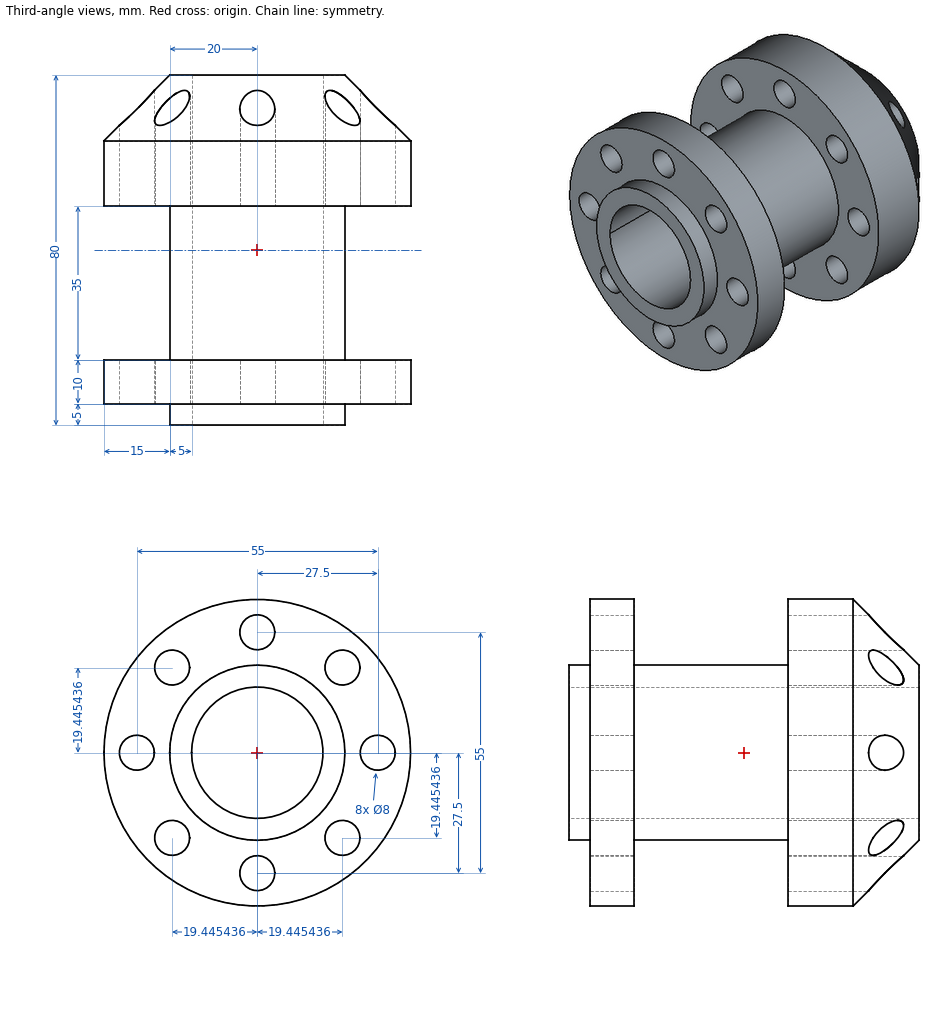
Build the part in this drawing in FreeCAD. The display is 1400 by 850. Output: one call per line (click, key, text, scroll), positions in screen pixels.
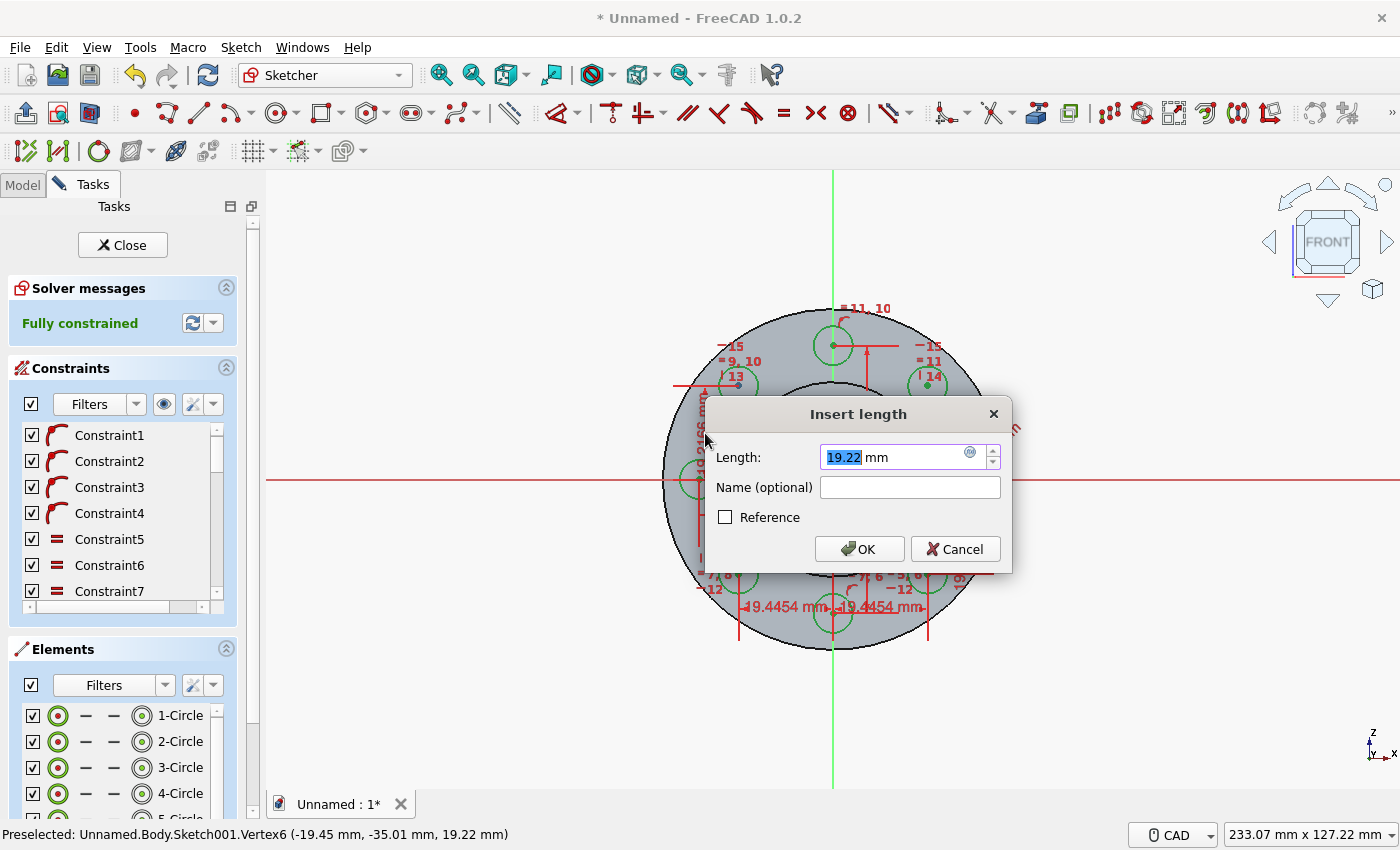
text(19.445436)
key(Return)
key(Escape)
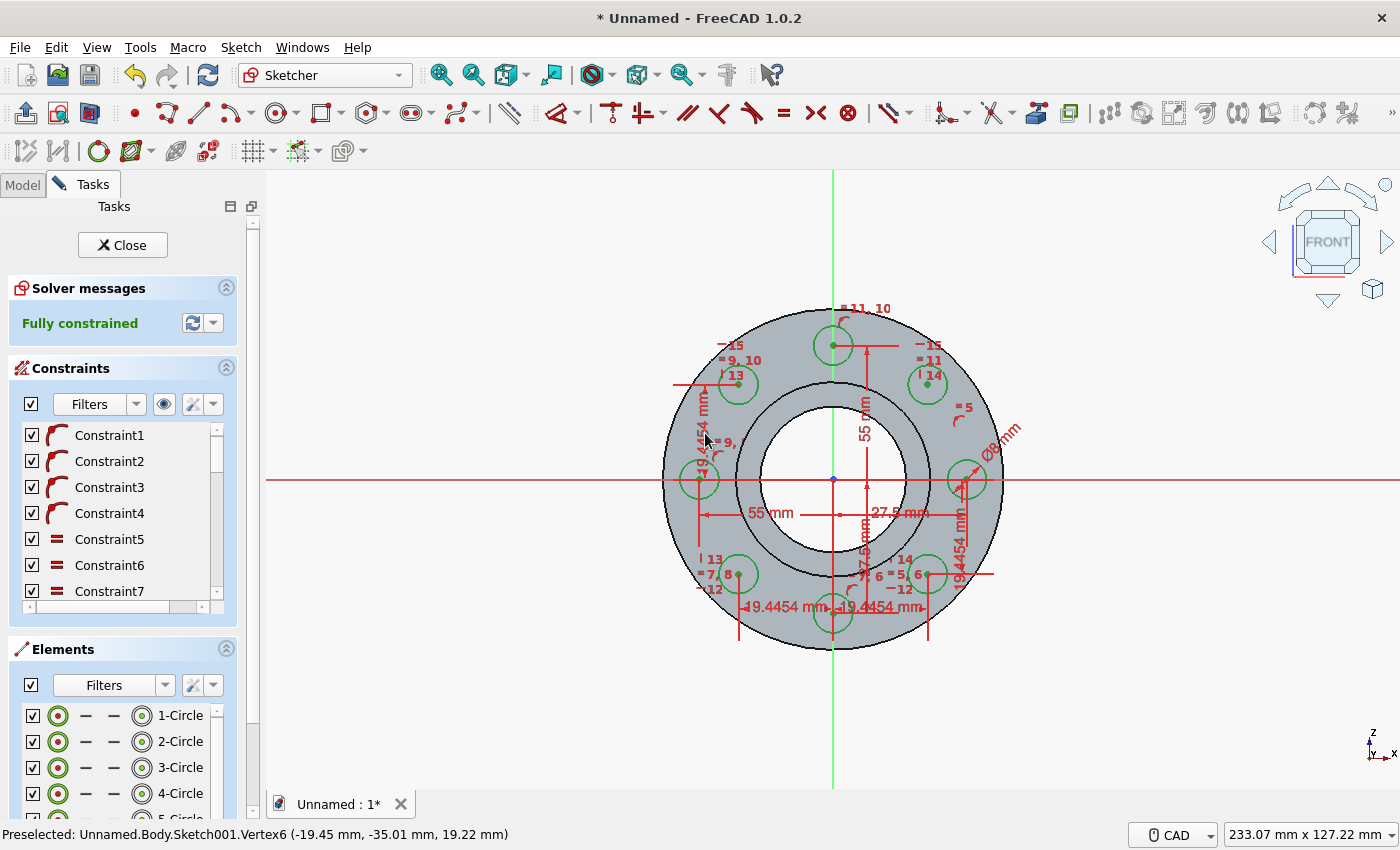
click(123, 245)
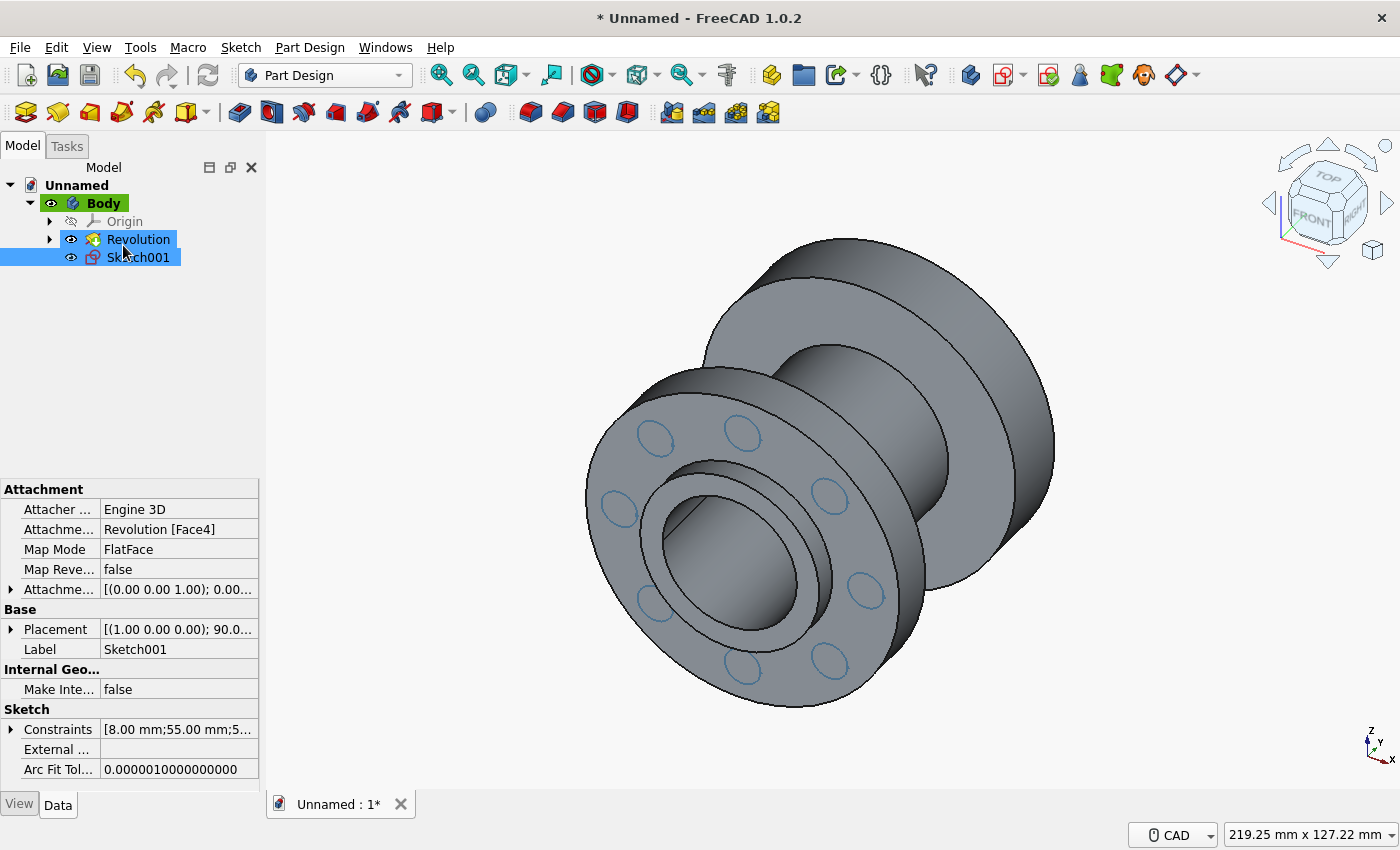
click(240, 112)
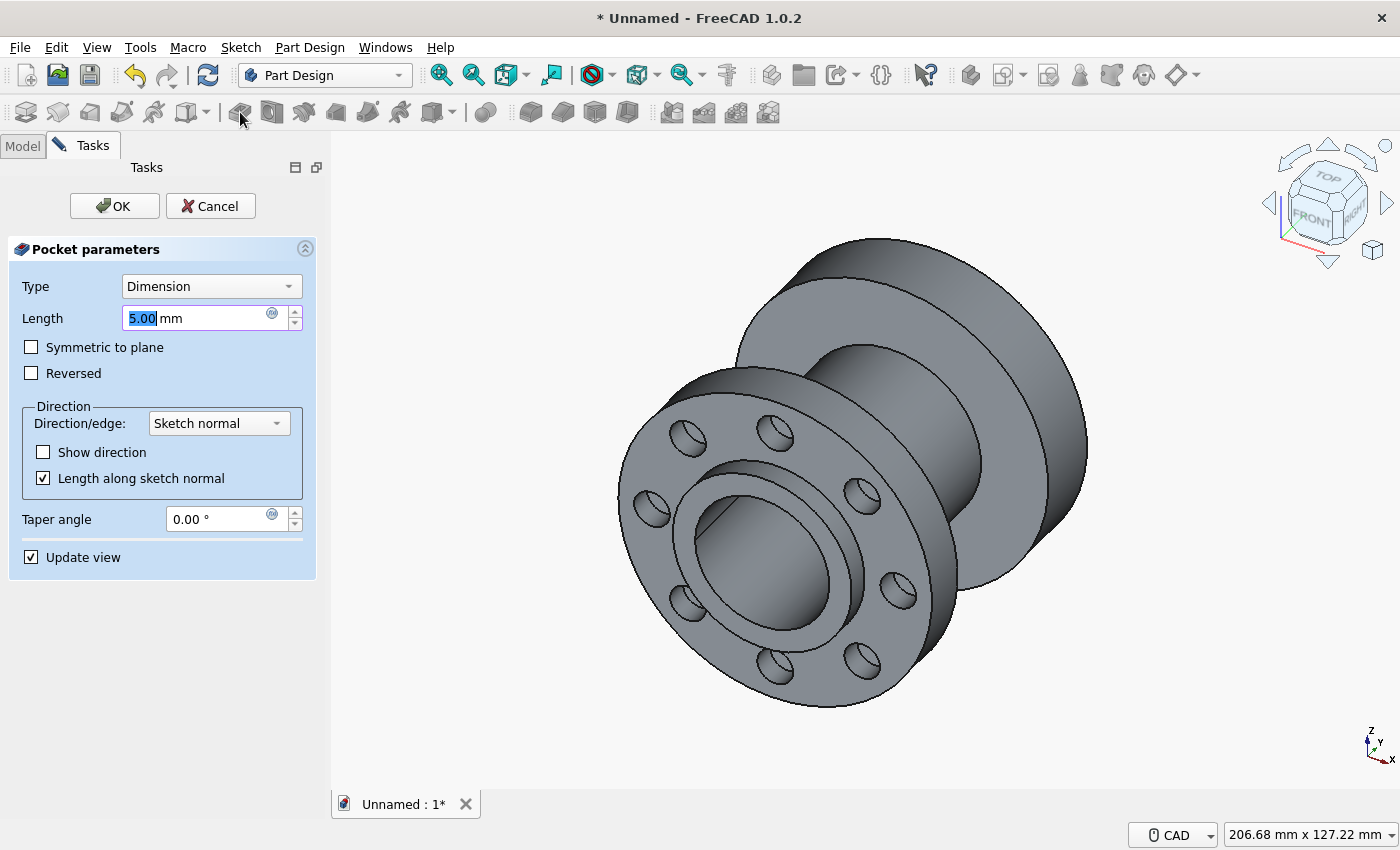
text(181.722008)
key(Tab)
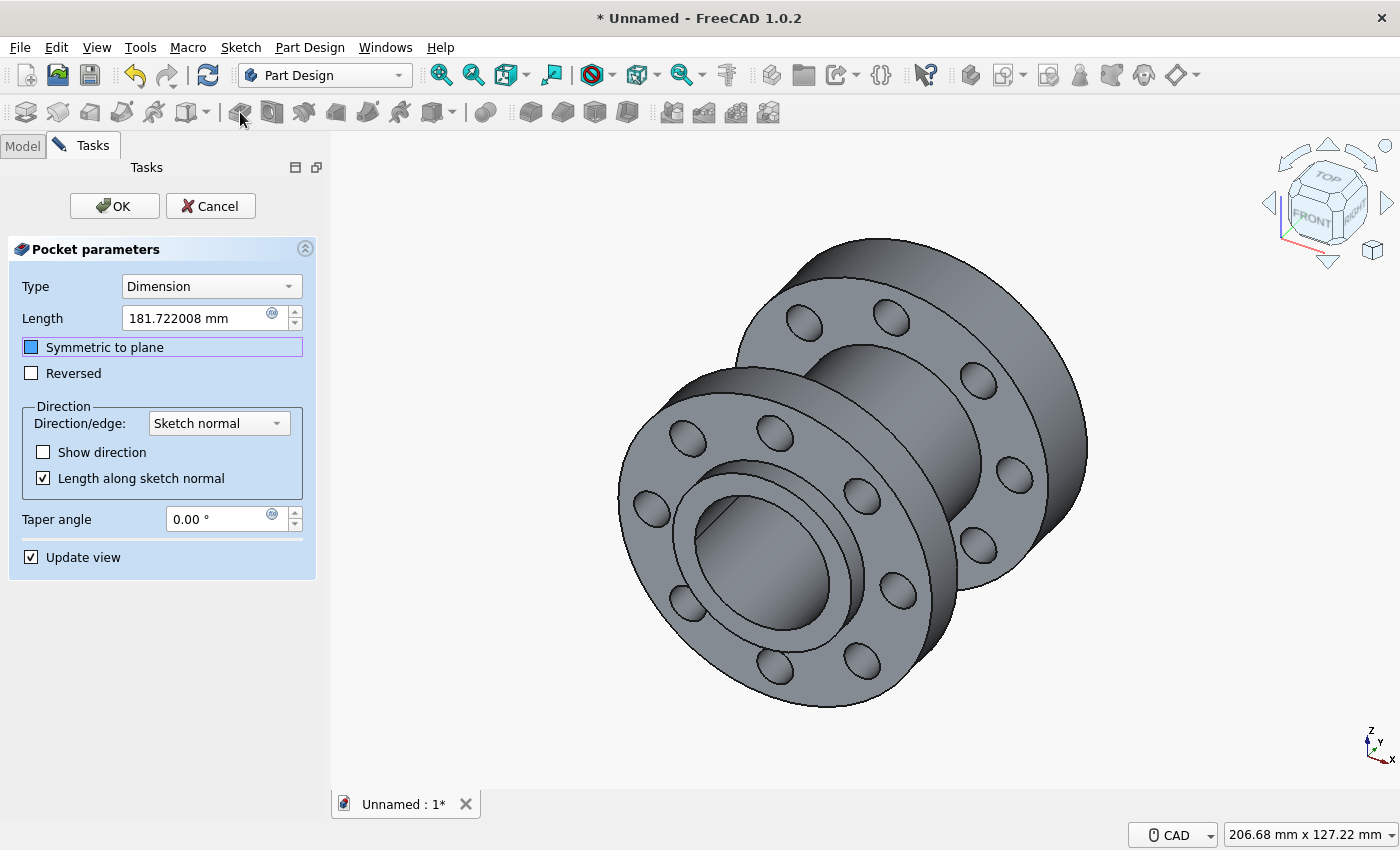
click(30, 347)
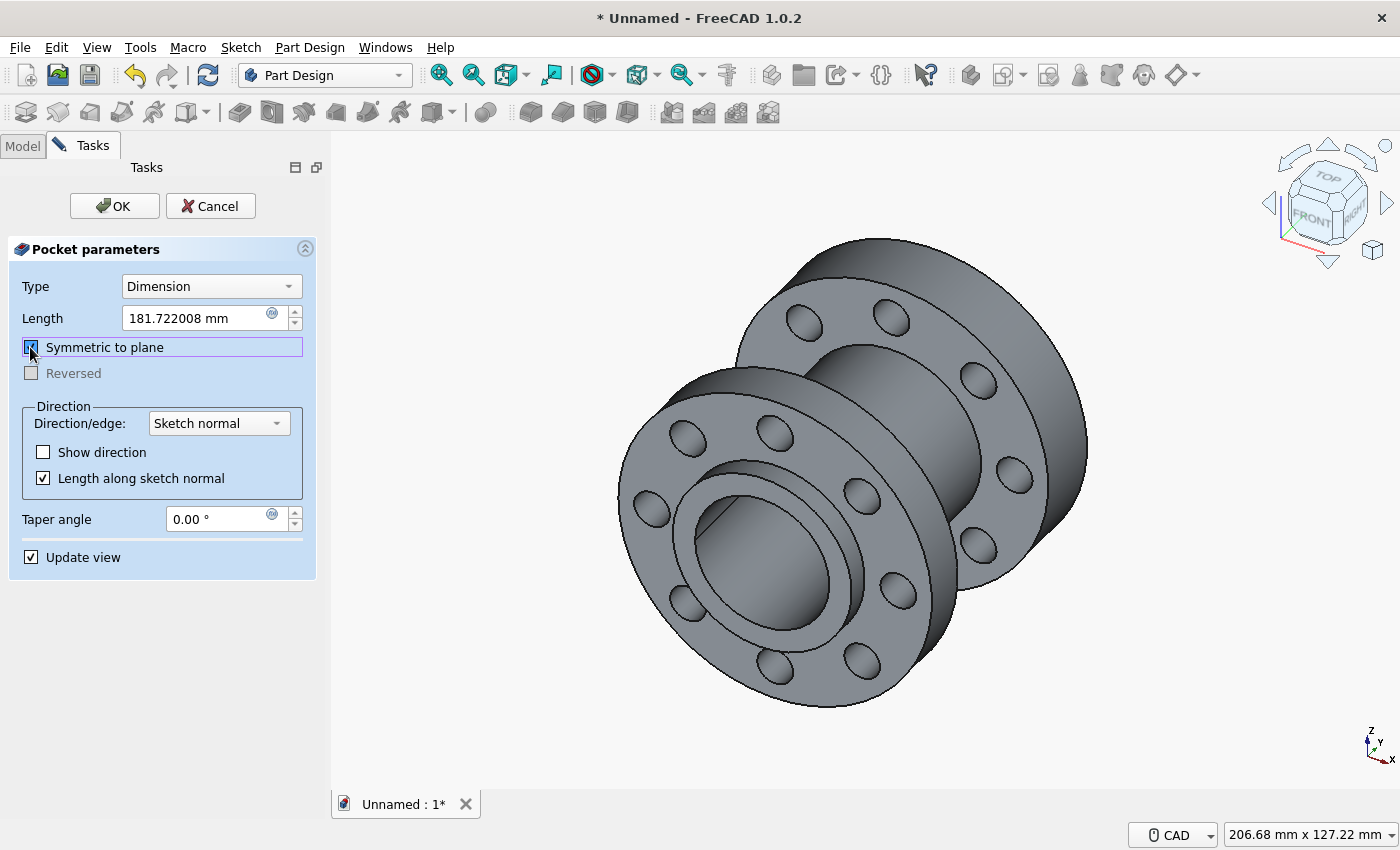
click(115, 206)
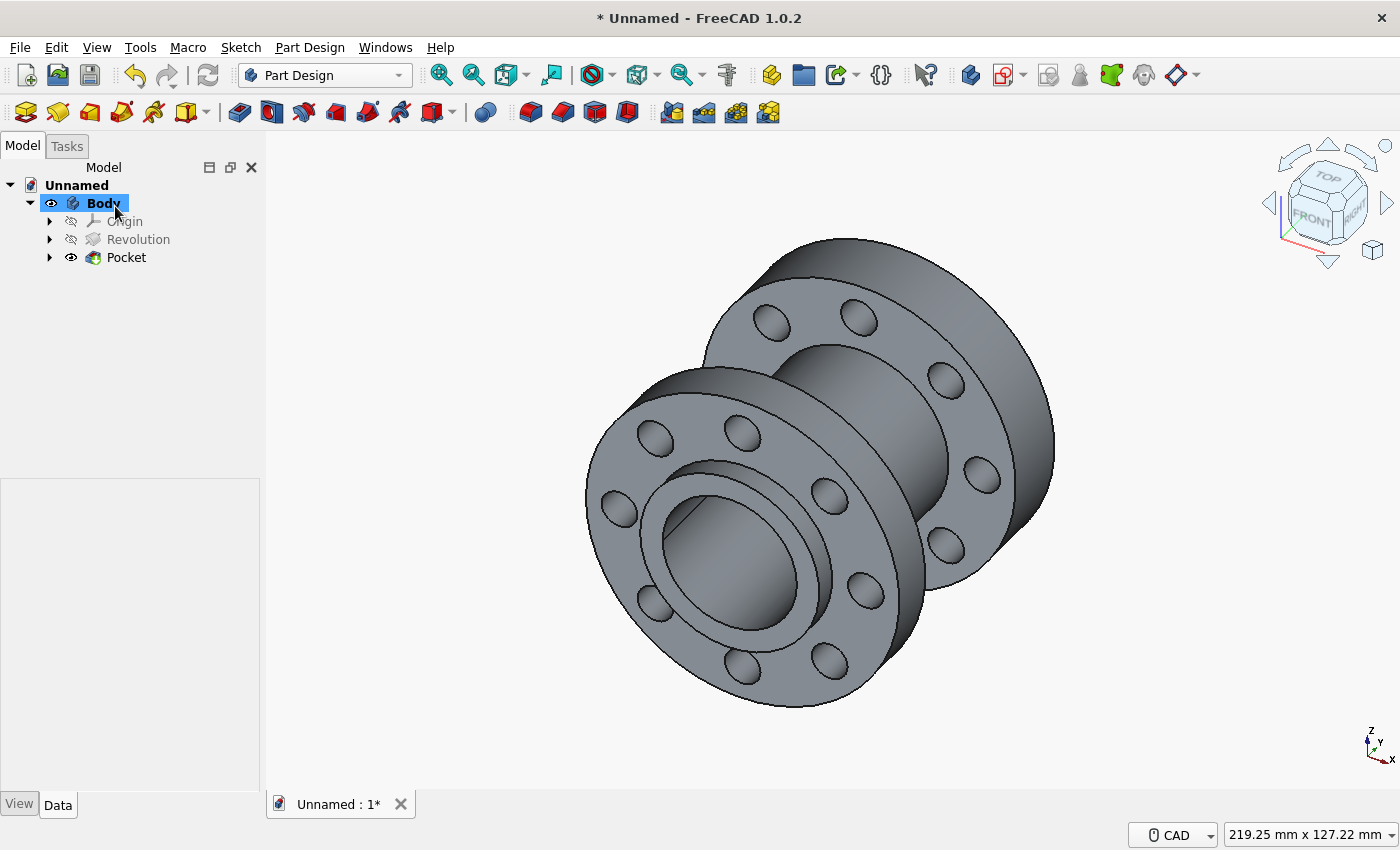
key(0)